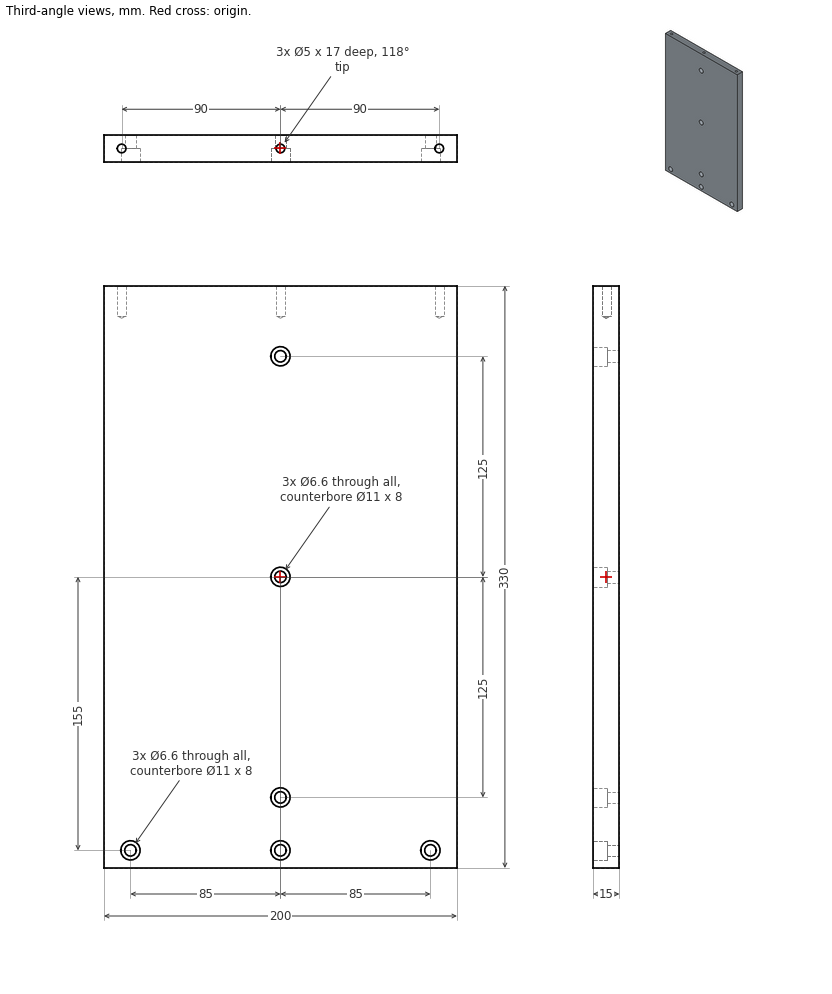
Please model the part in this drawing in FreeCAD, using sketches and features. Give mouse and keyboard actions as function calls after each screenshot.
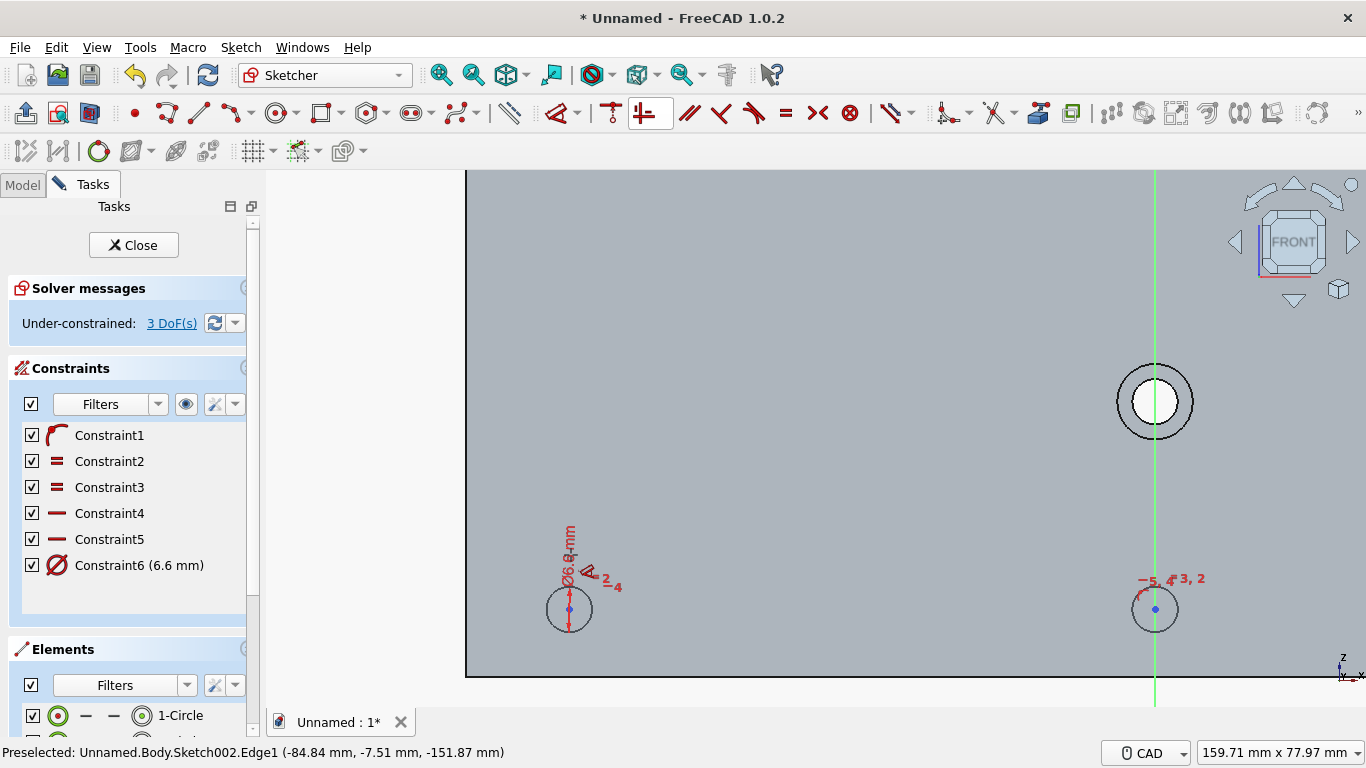
click(569, 609)
click(862, 643)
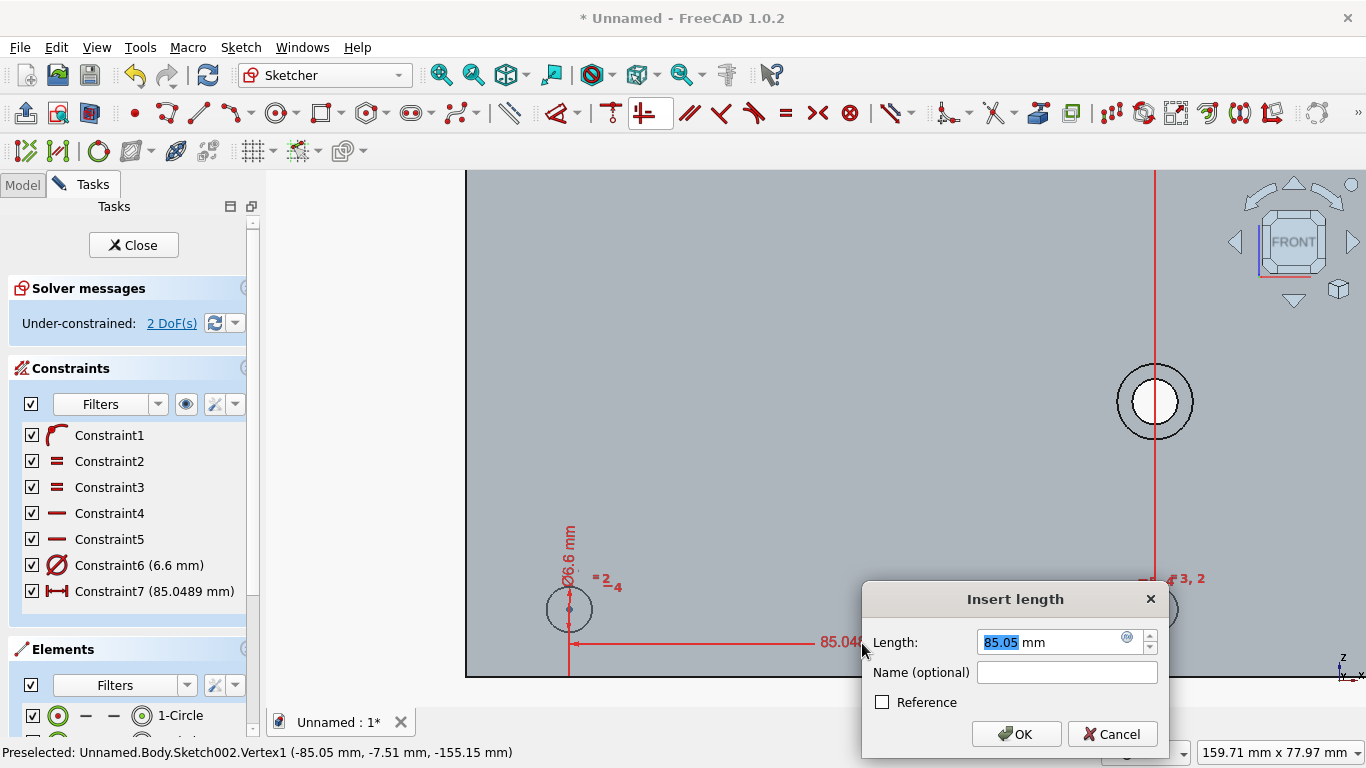
text(85)
key(Return)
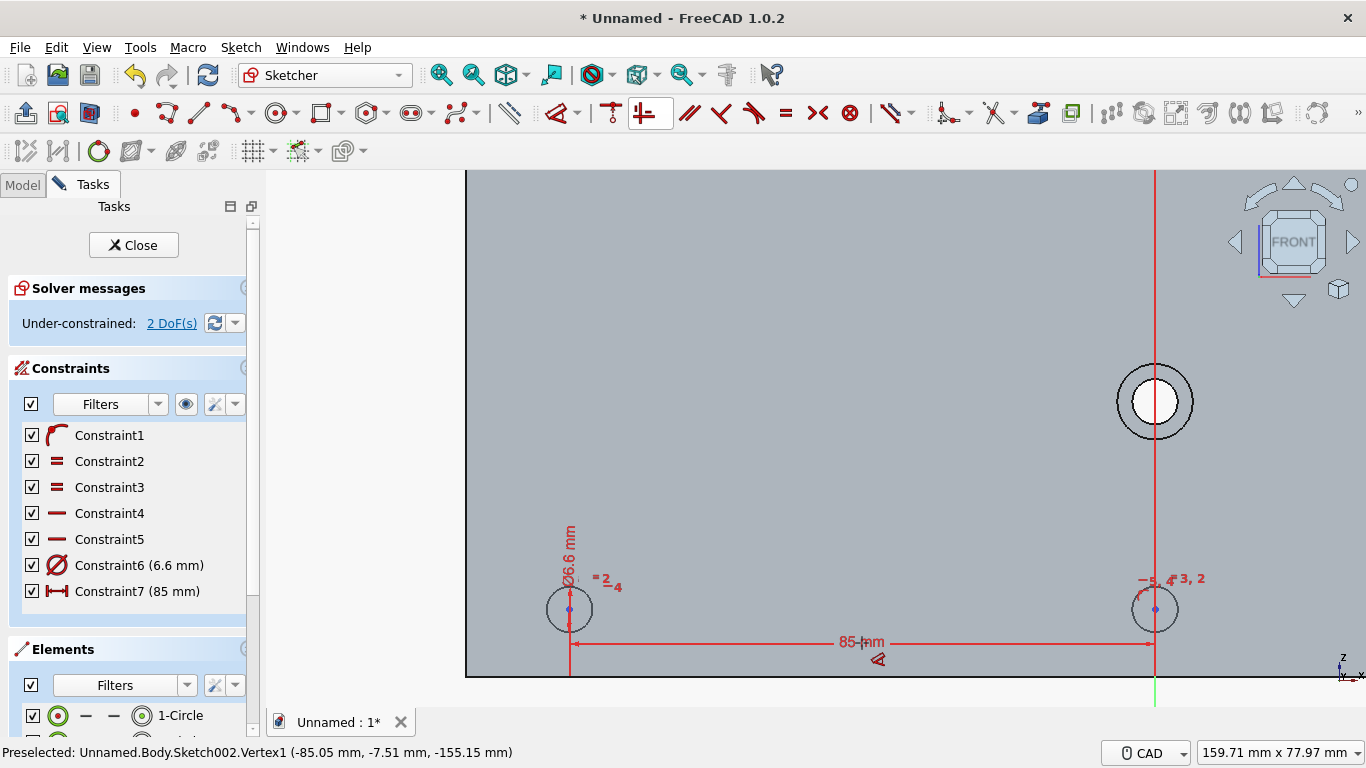
scroll(572, 590, down, 6)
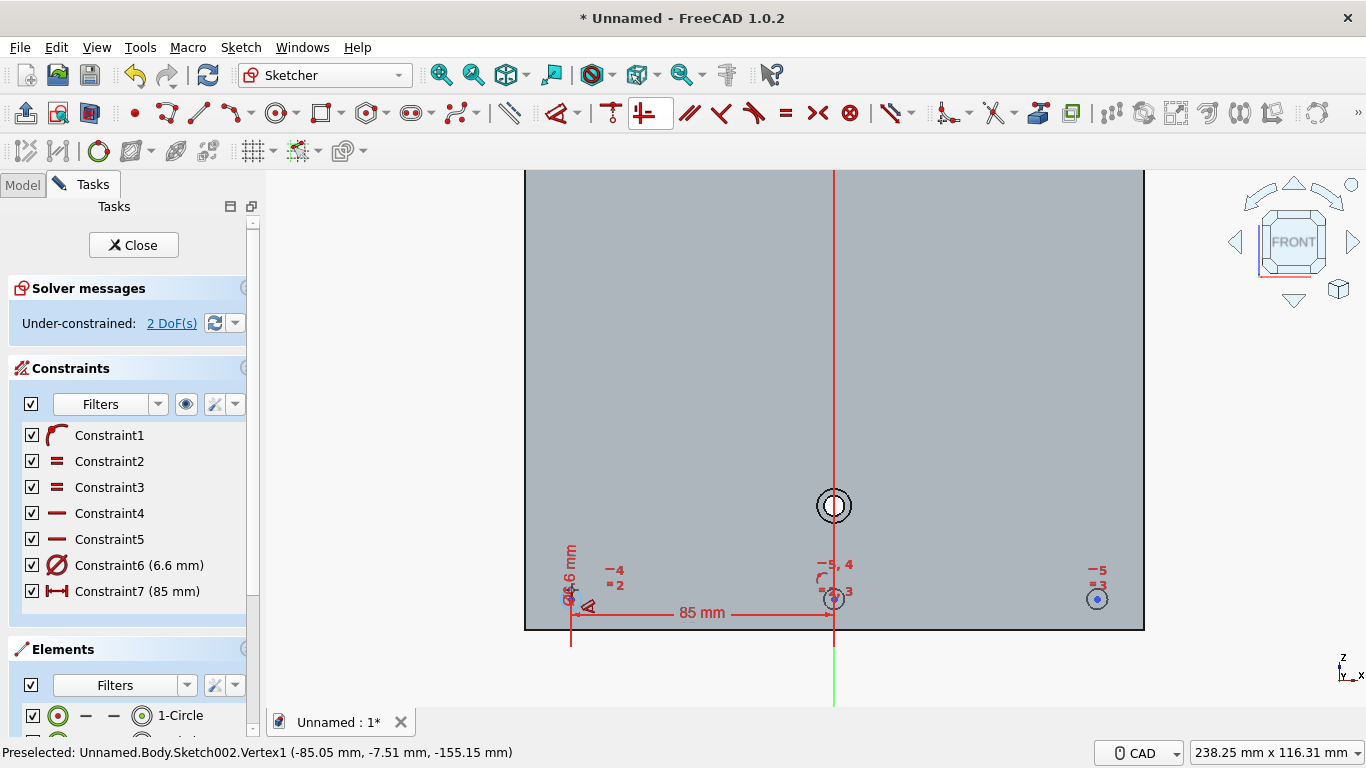
click(924, 596)
click(836, 241)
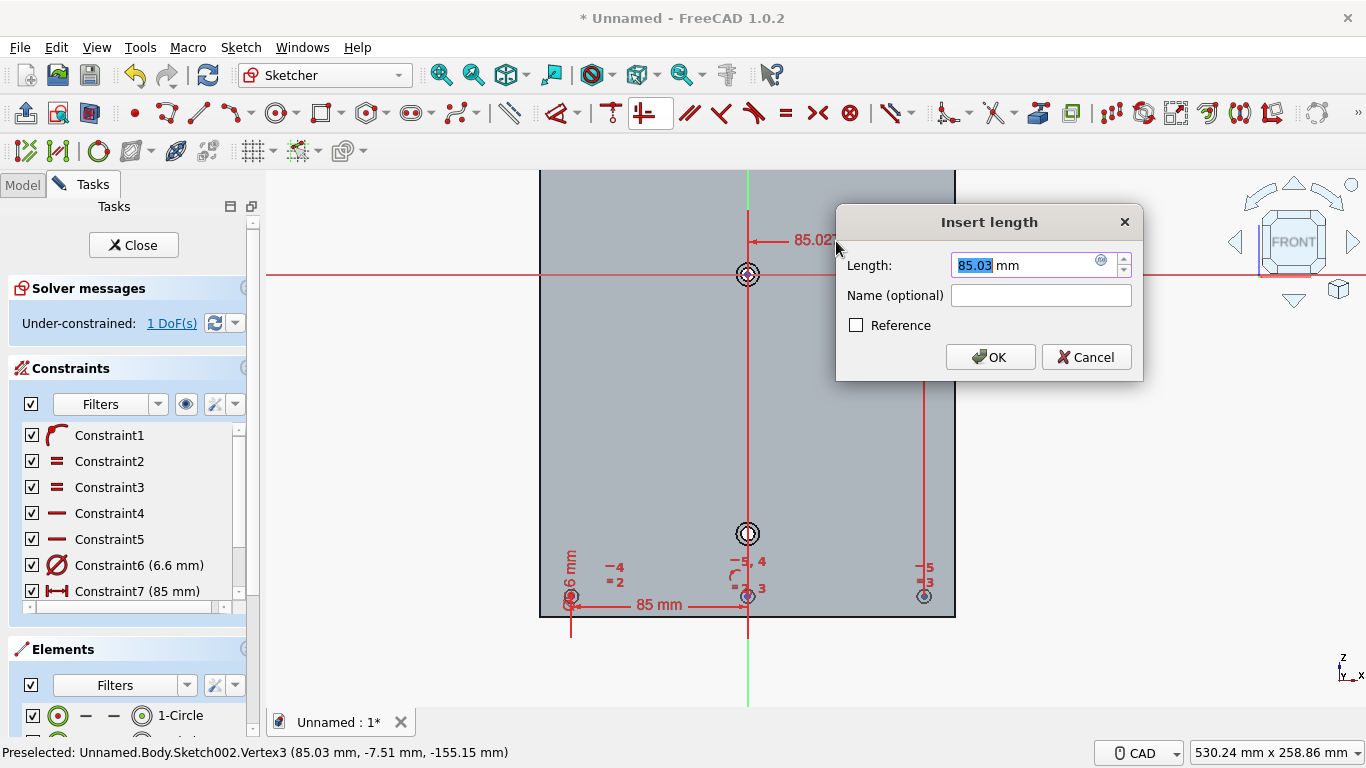
text(85)
key(Return)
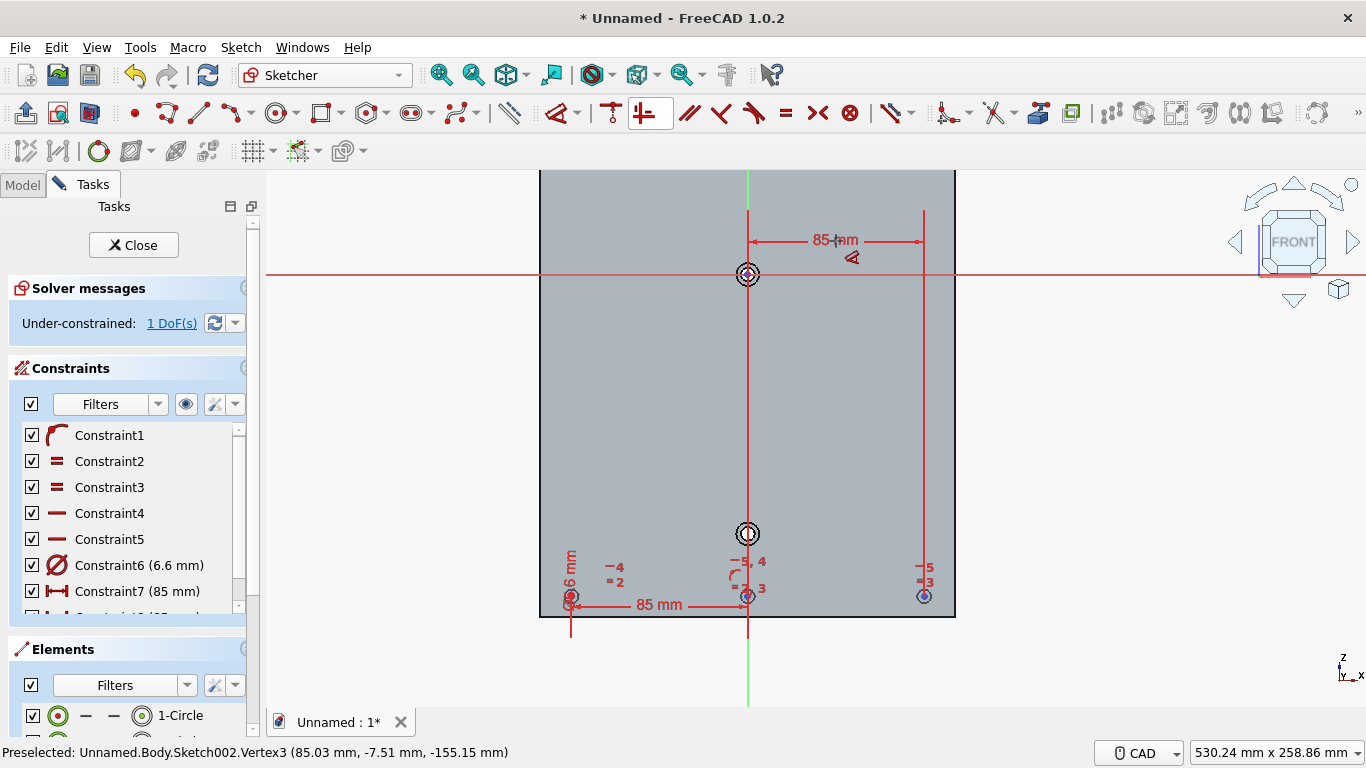
click(571, 596)
click(537, 435)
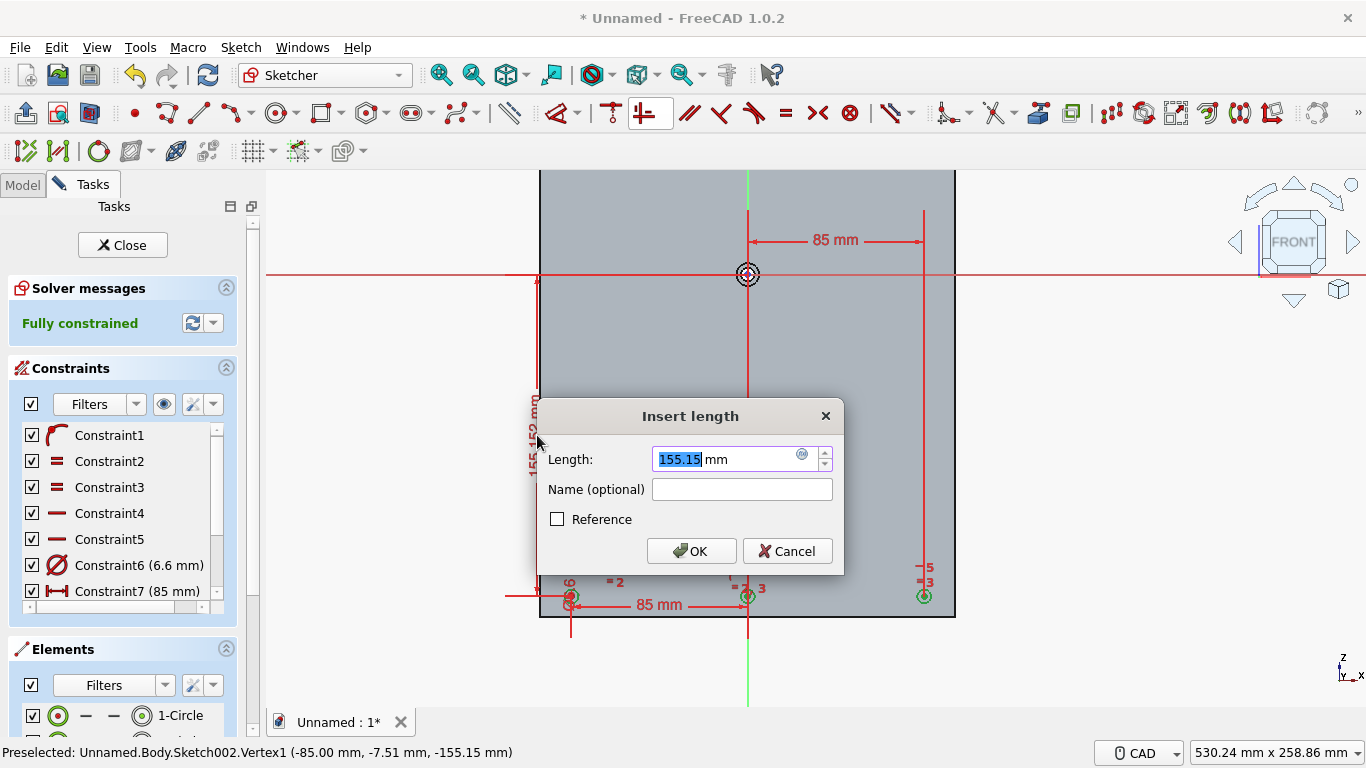
text(155)
key(Return)
key(Escape)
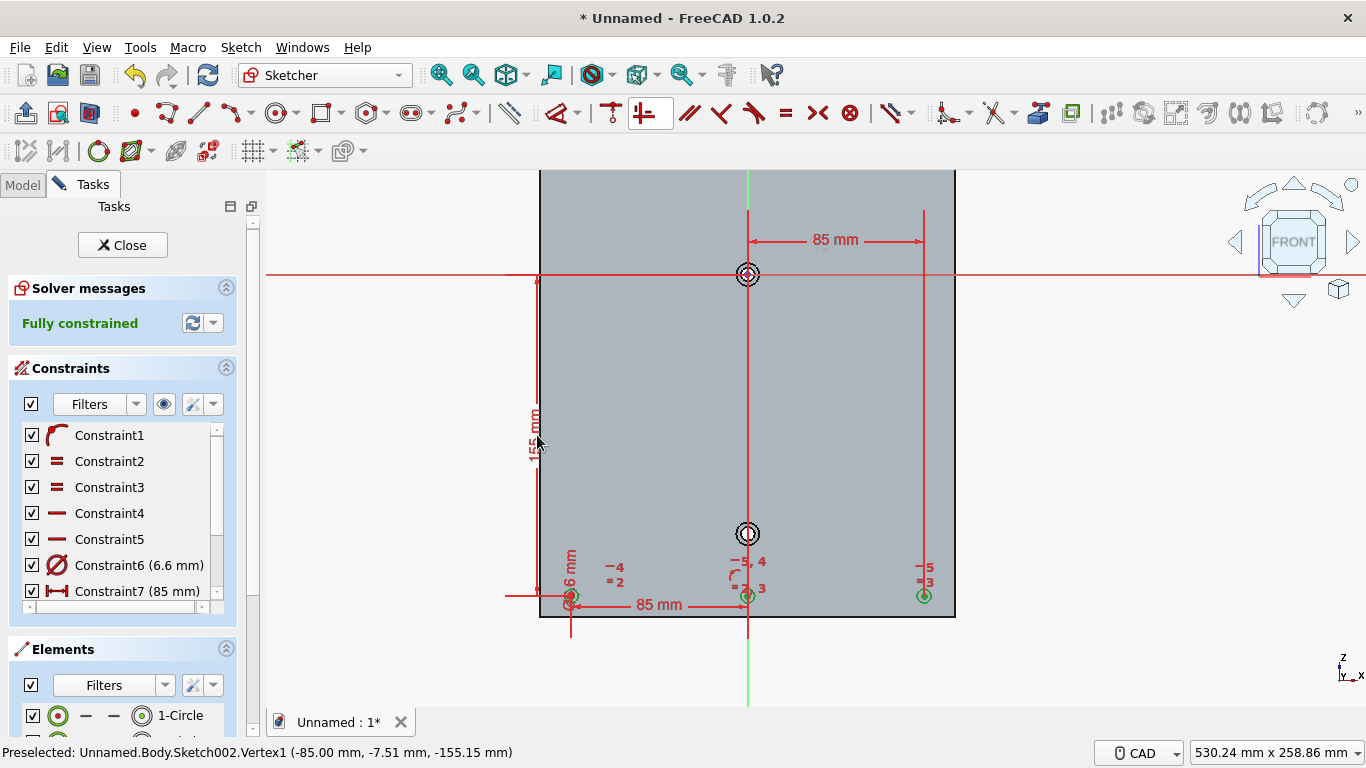
click(123, 245)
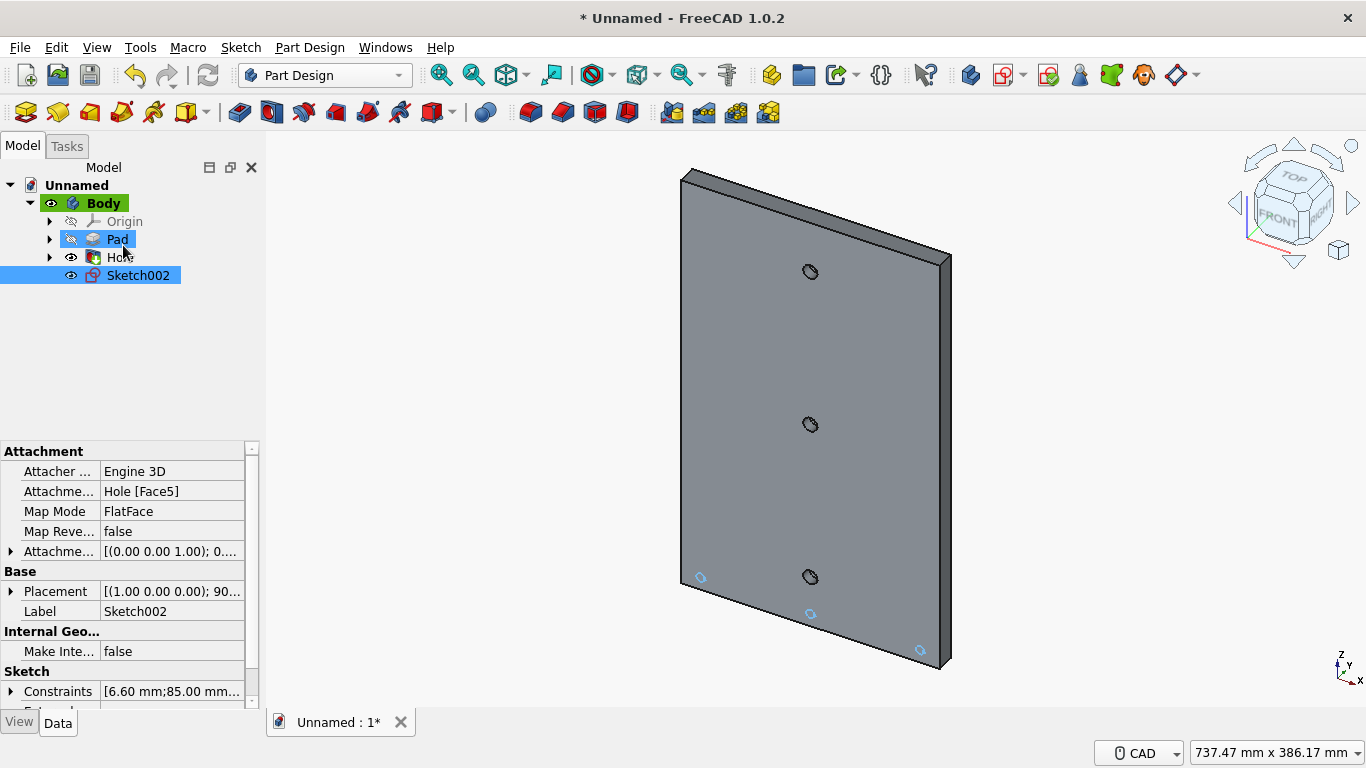
click(272, 112)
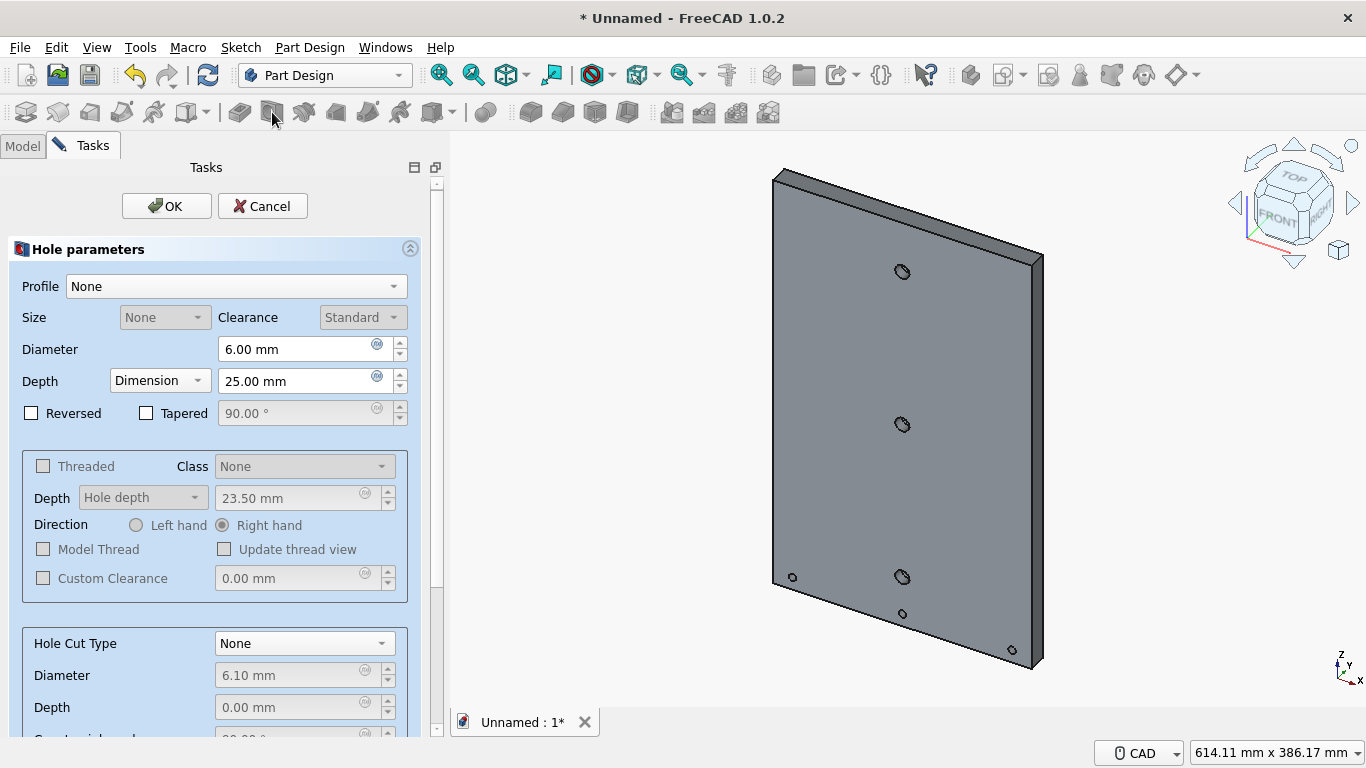
triple_click(305, 349)